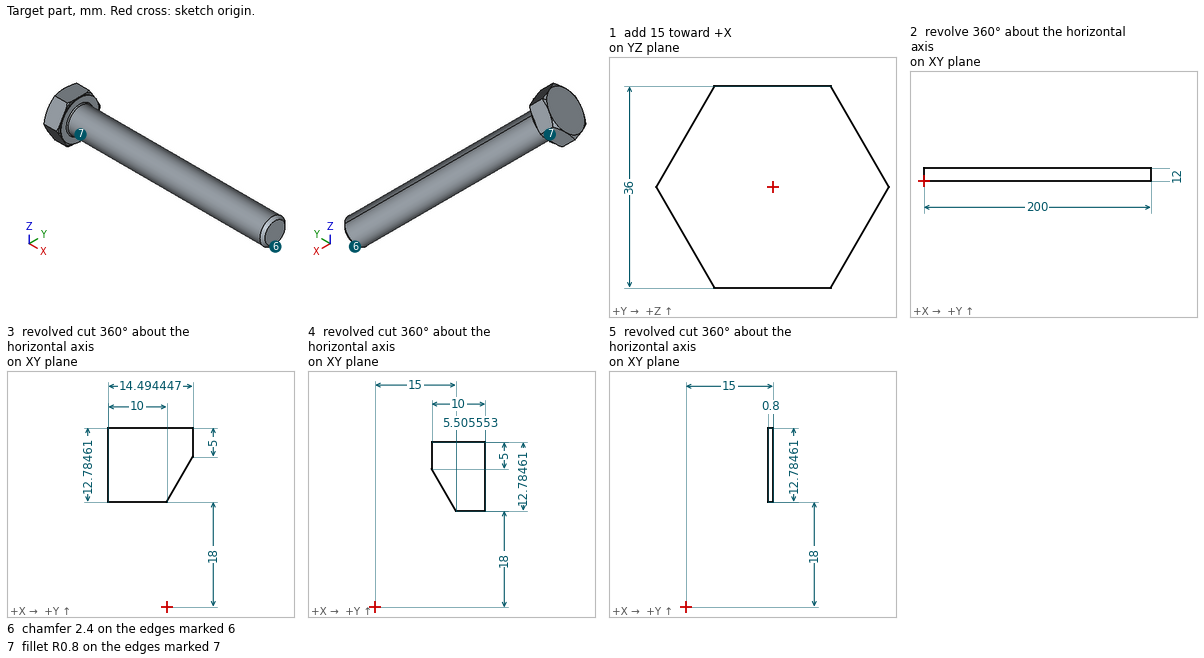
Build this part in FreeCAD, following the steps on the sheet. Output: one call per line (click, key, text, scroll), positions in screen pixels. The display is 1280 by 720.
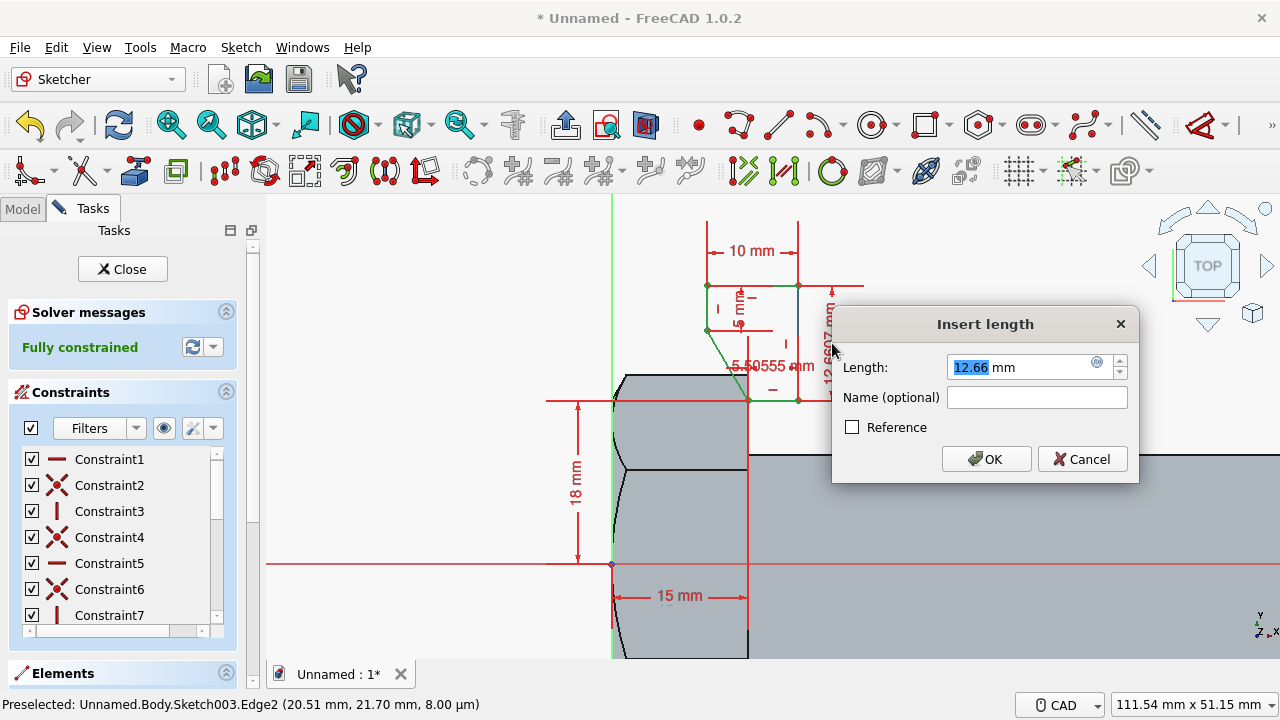
text(12.78461)
key(Return)
key(Escape)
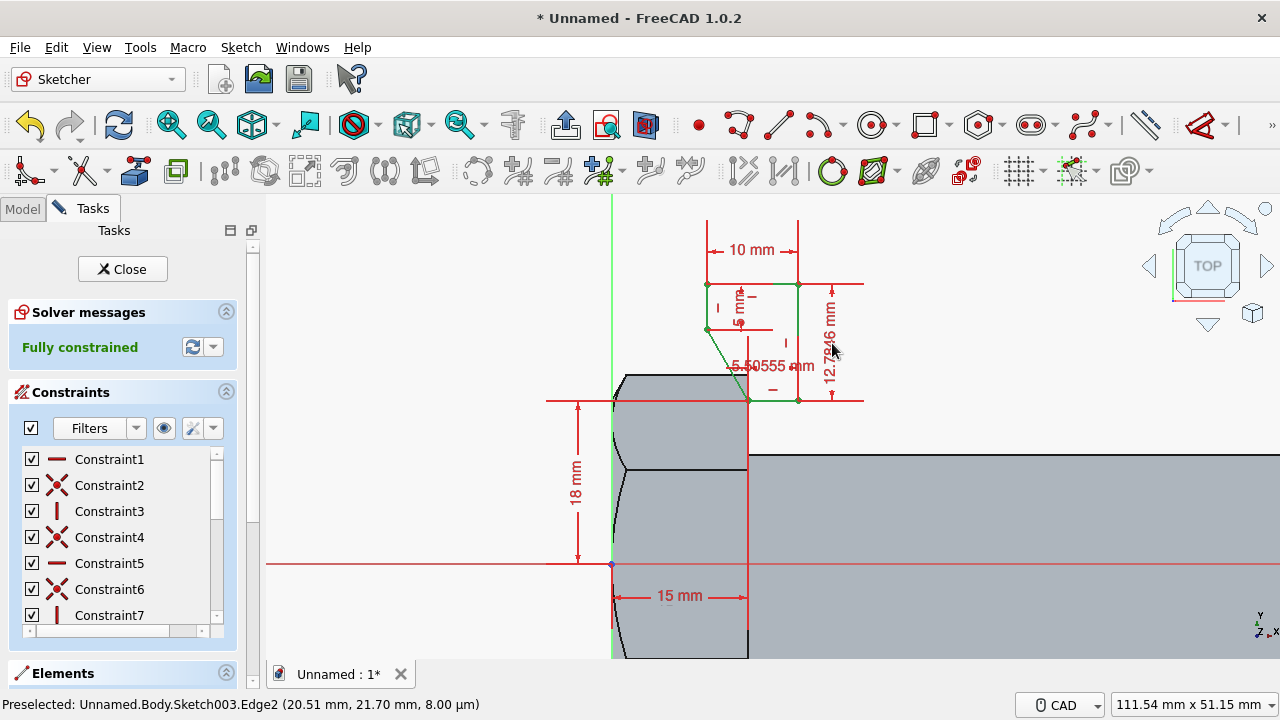
click(123, 269)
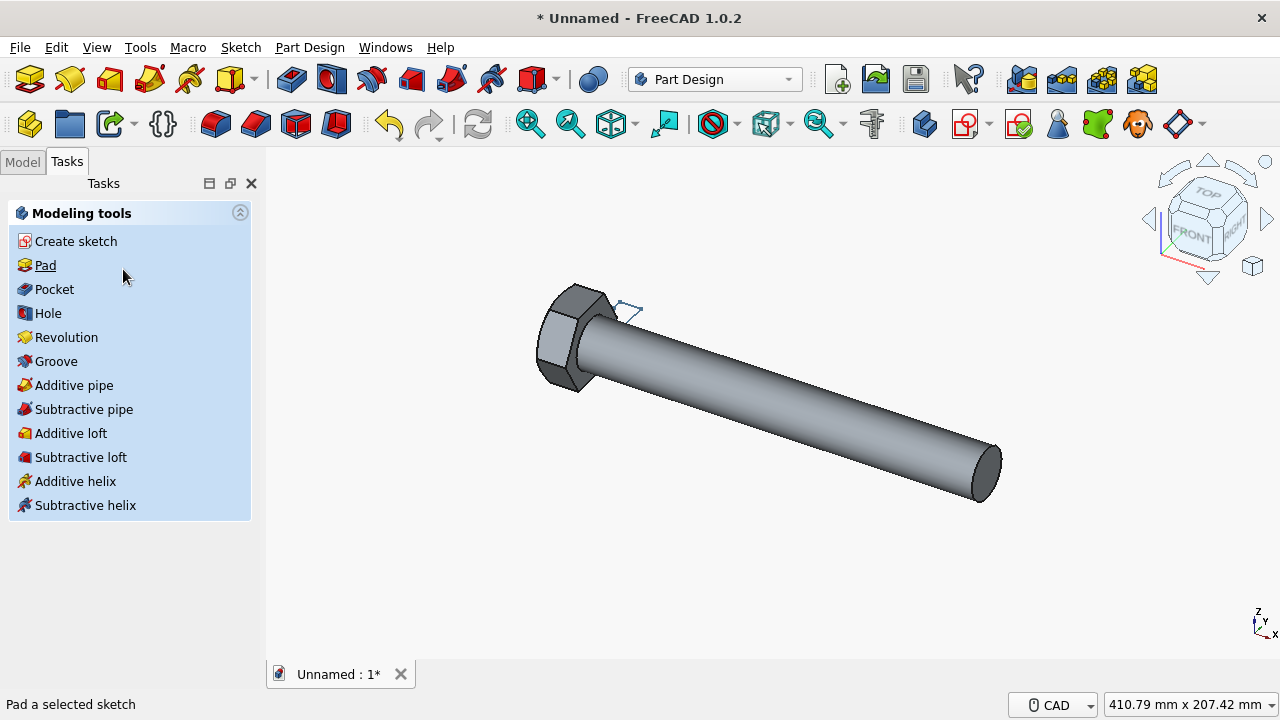
click(372, 80)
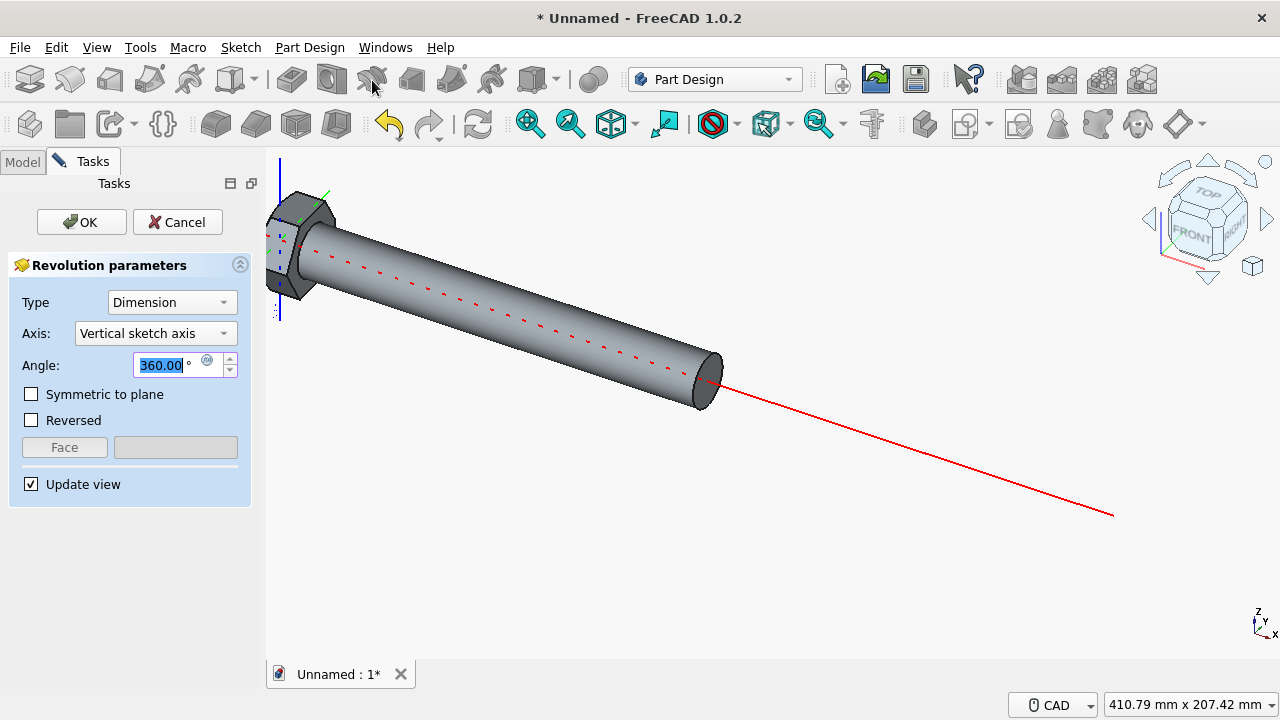
click(156, 334)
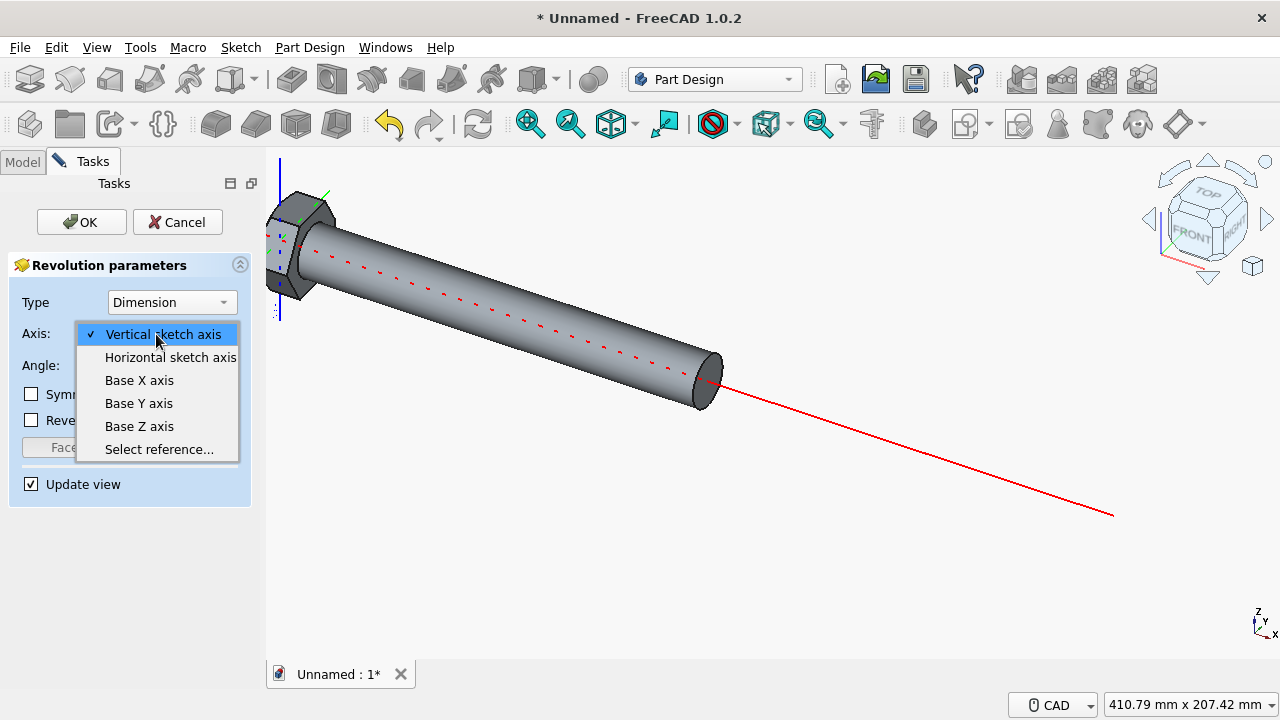
click(156, 358)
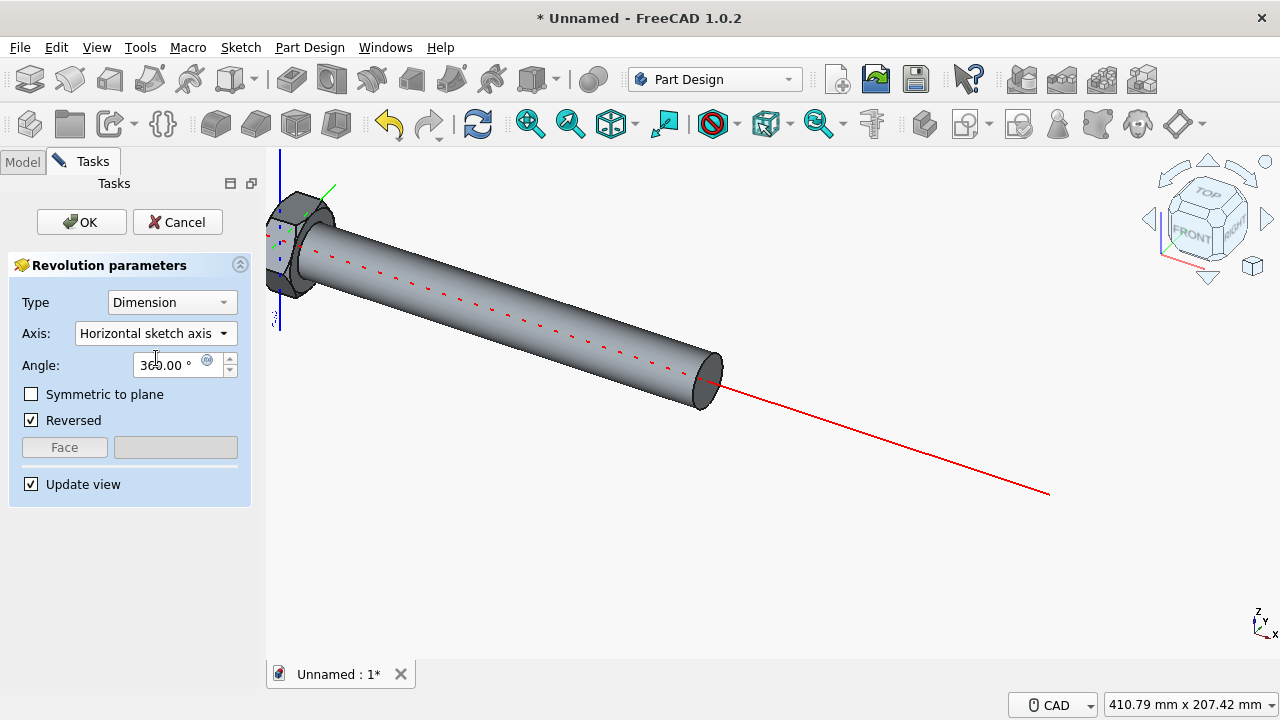
click(82, 222)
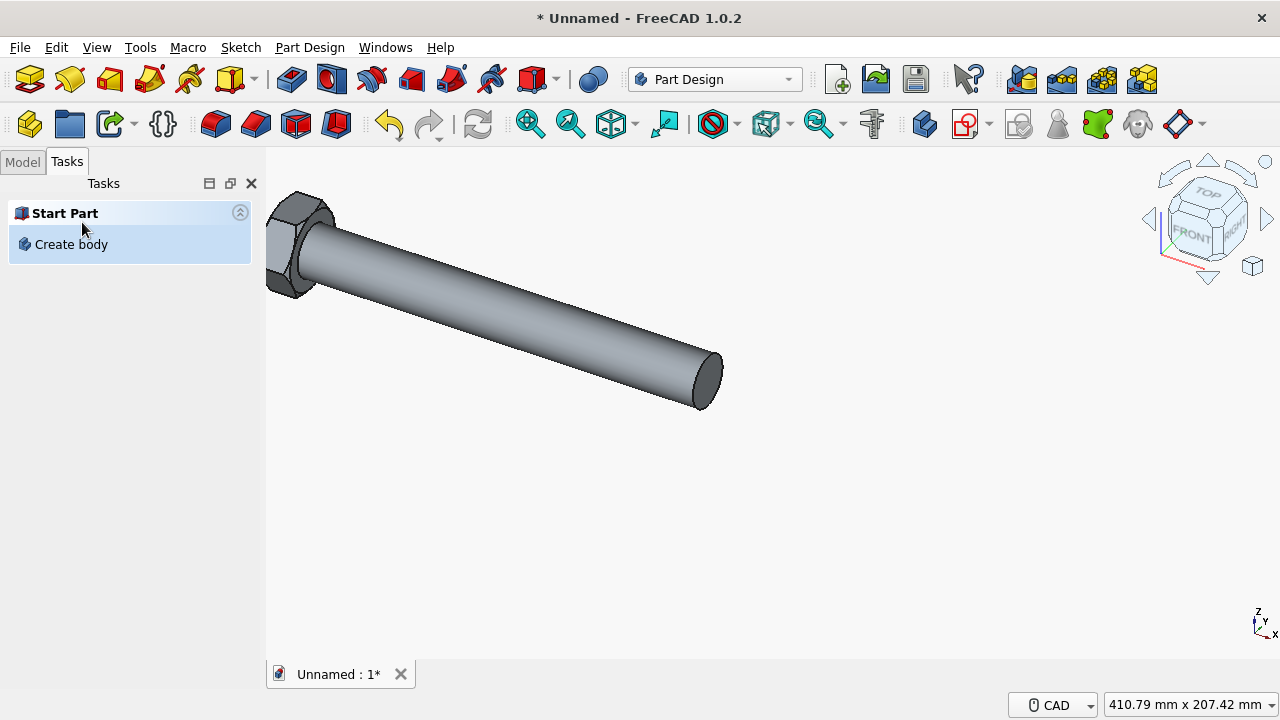
key(v)
key(f)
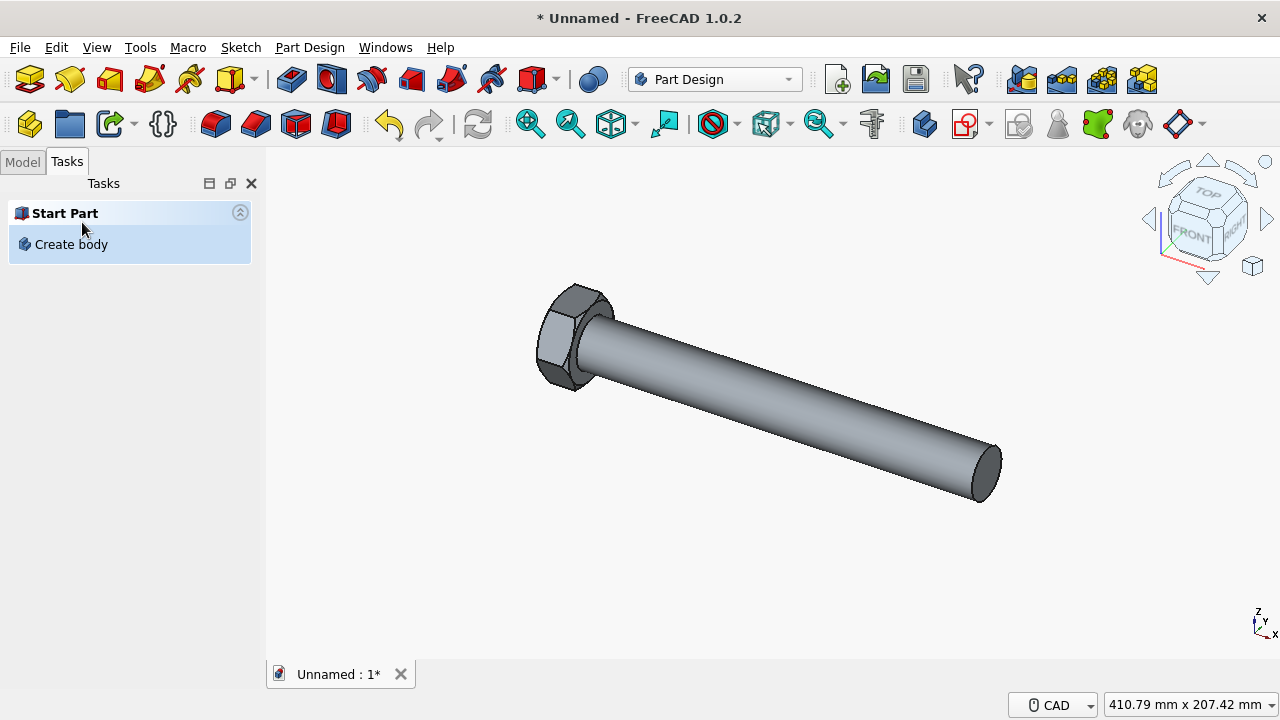
click(966, 124)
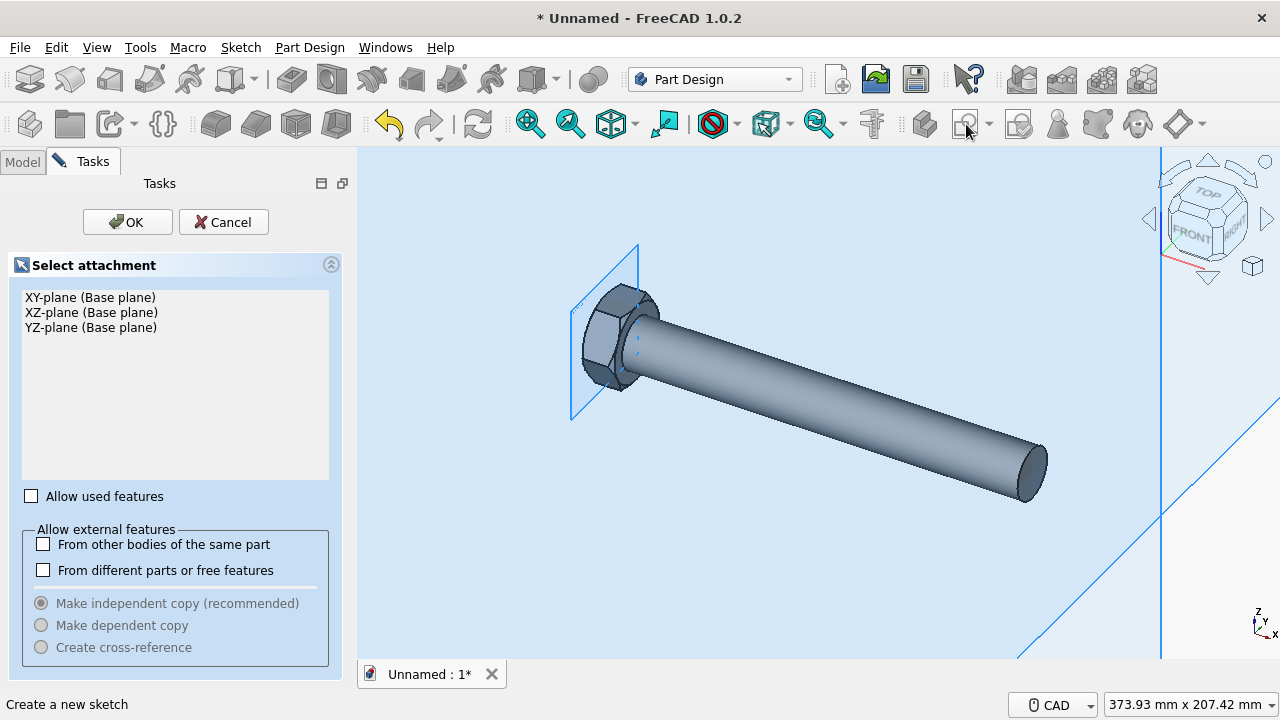
click(82, 298)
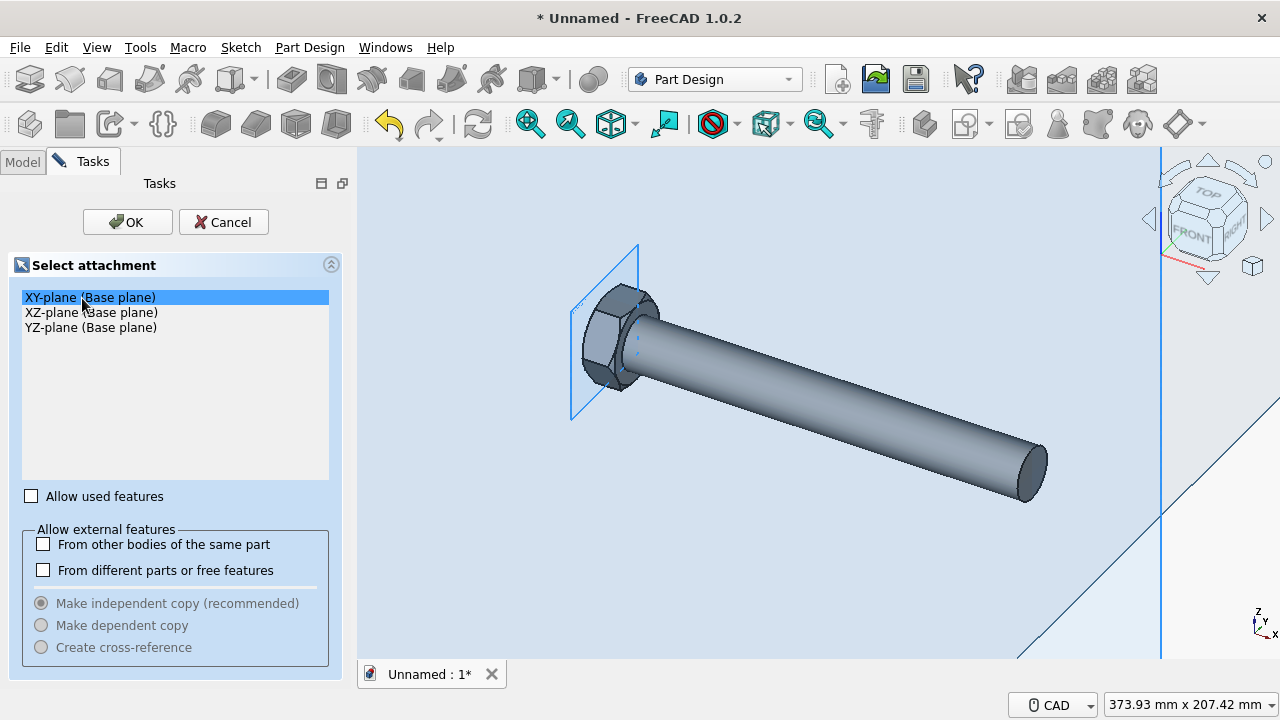
click(128, 222)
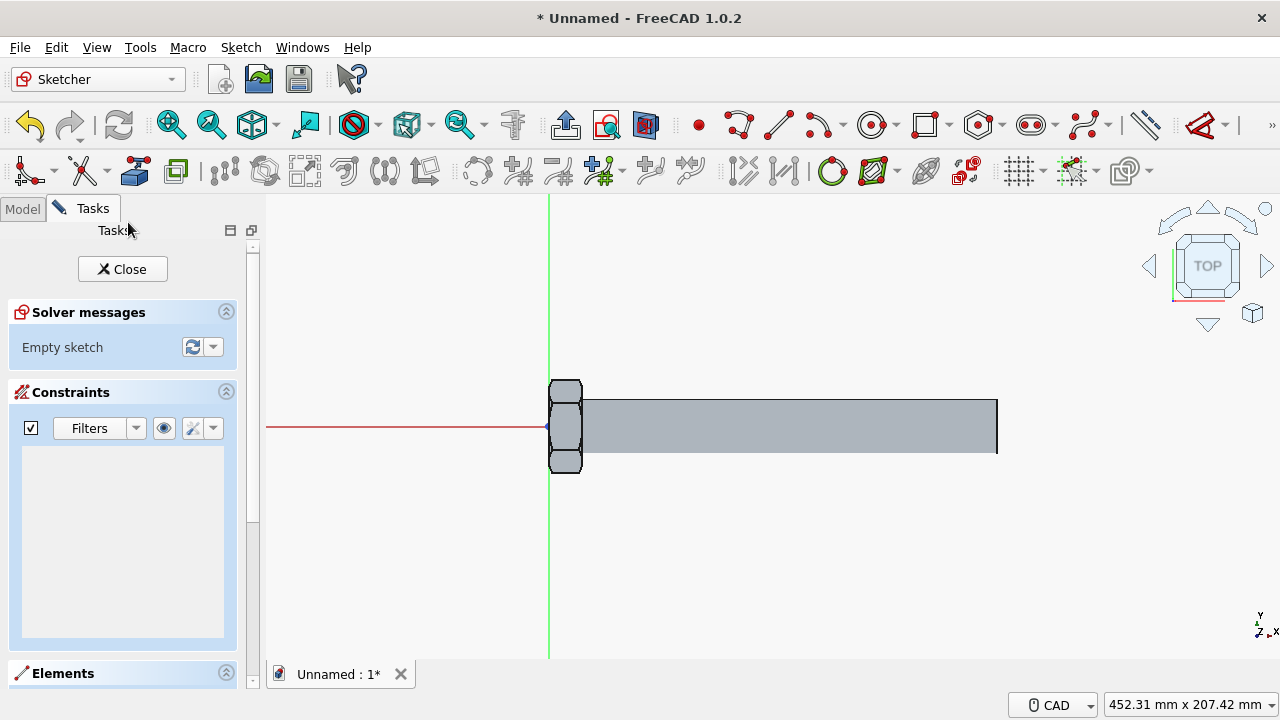
click(646, 126)